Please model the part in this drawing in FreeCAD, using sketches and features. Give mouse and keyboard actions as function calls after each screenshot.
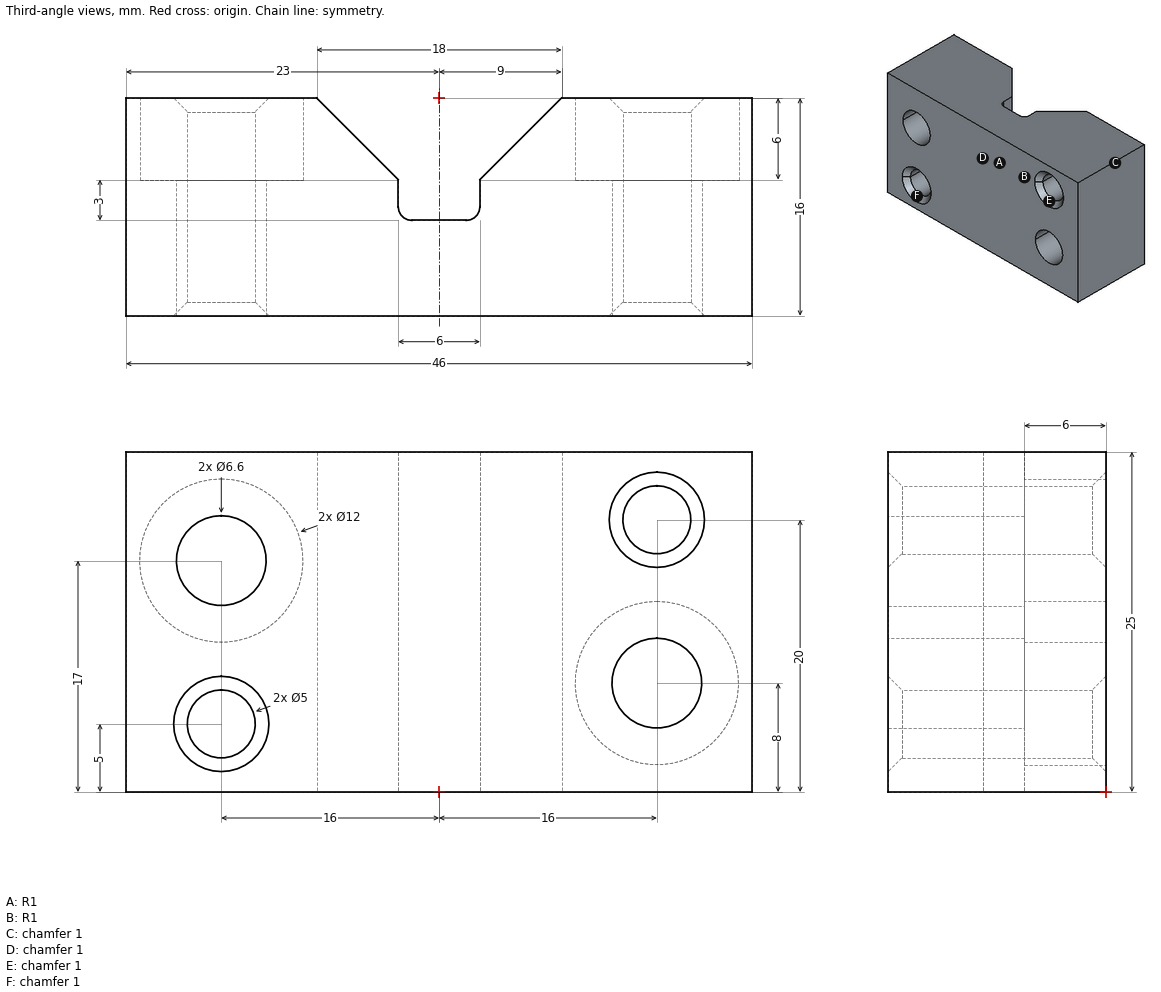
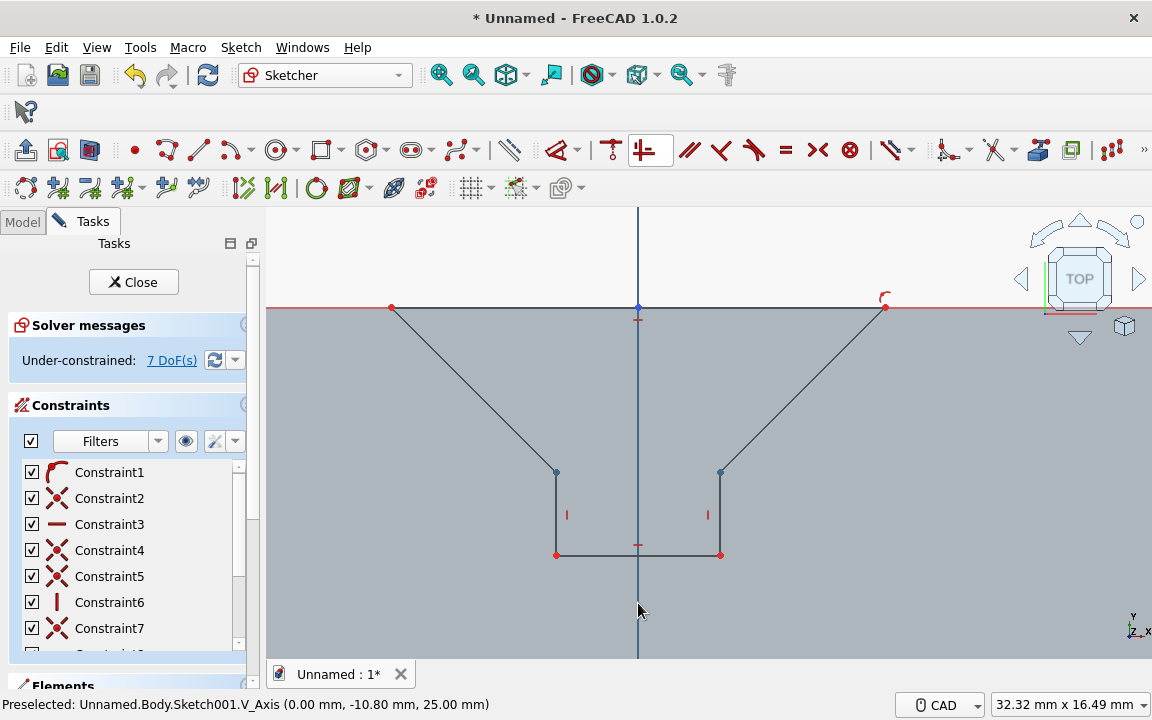
click(818, 150)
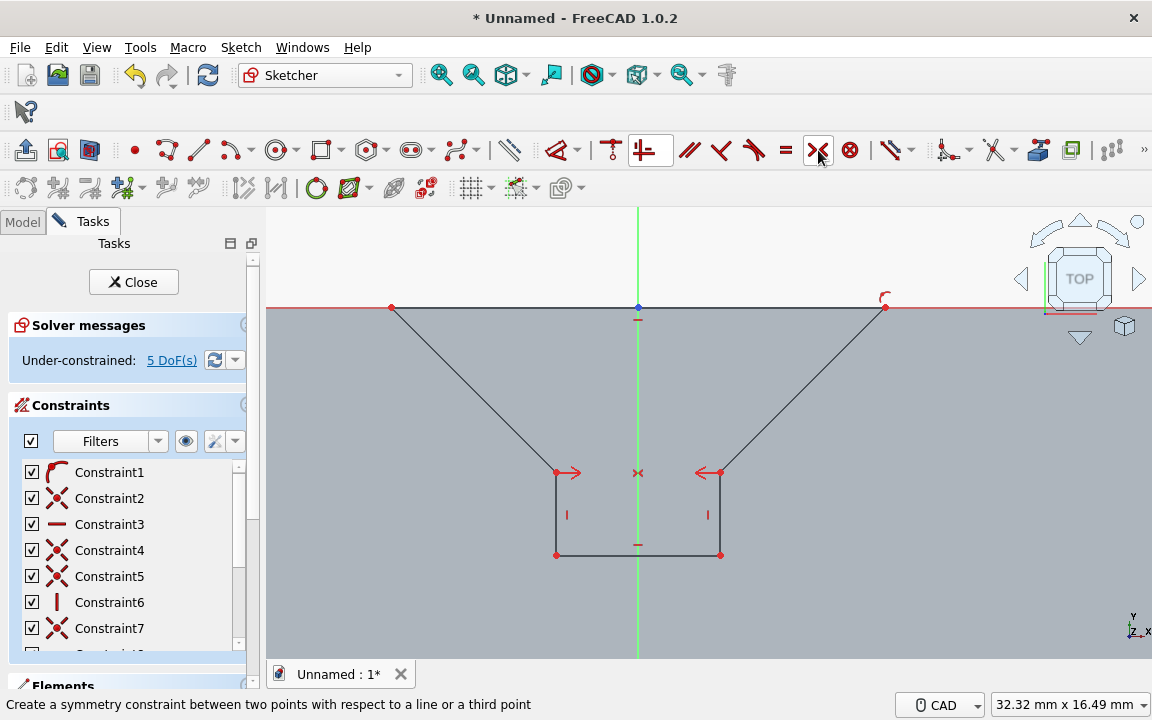
click(556, 498)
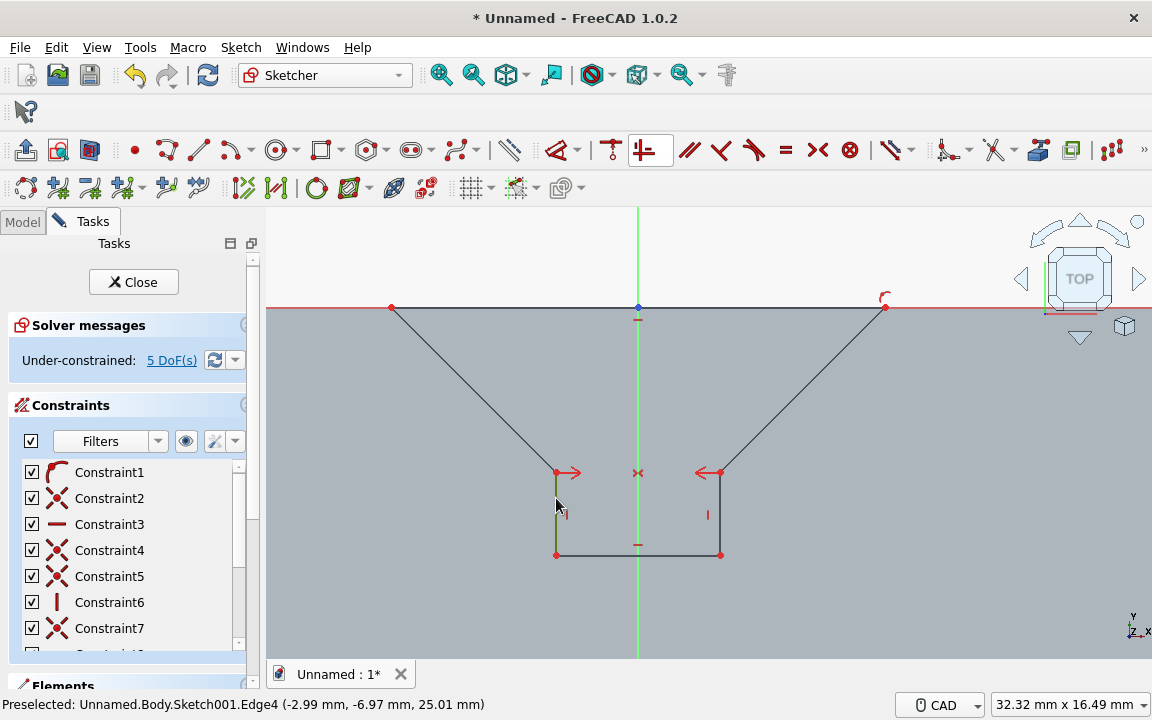
key(i)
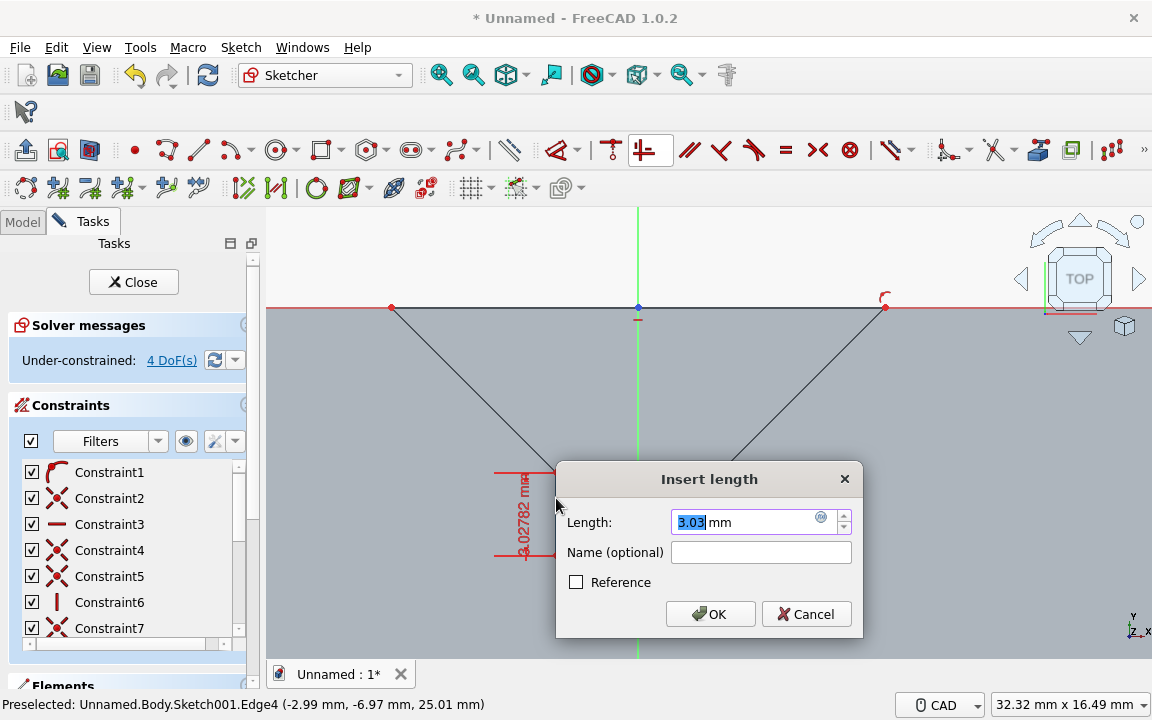
text(3)
key(Return)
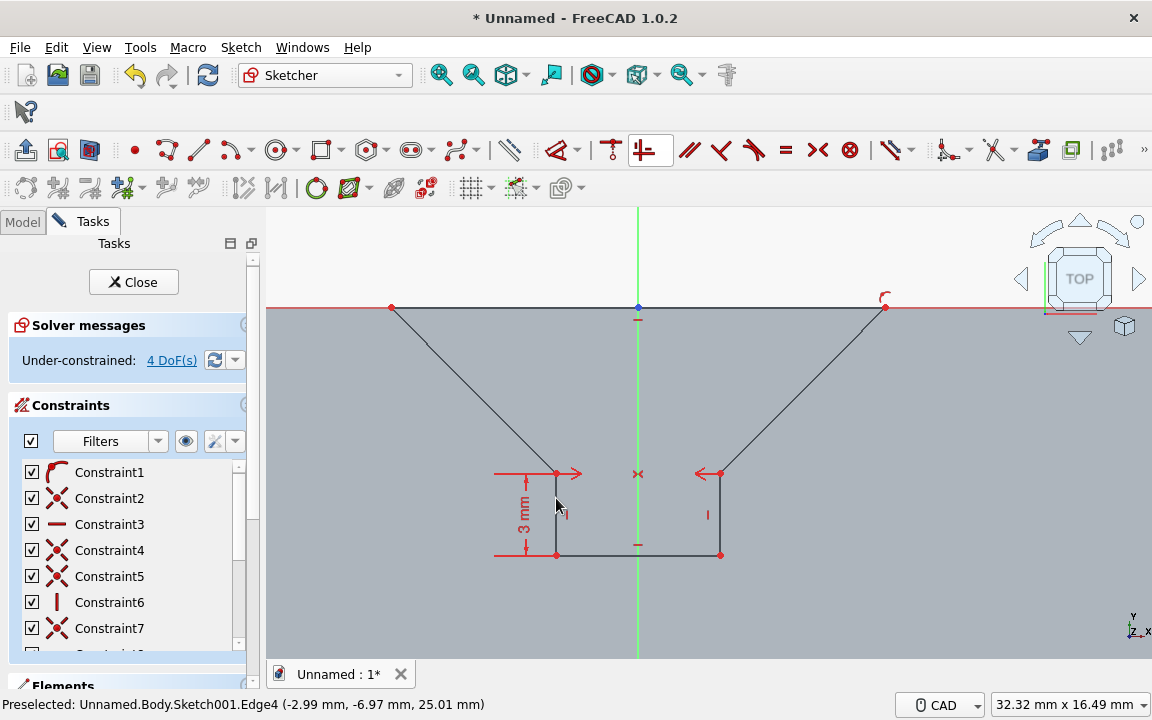
click(605, 556)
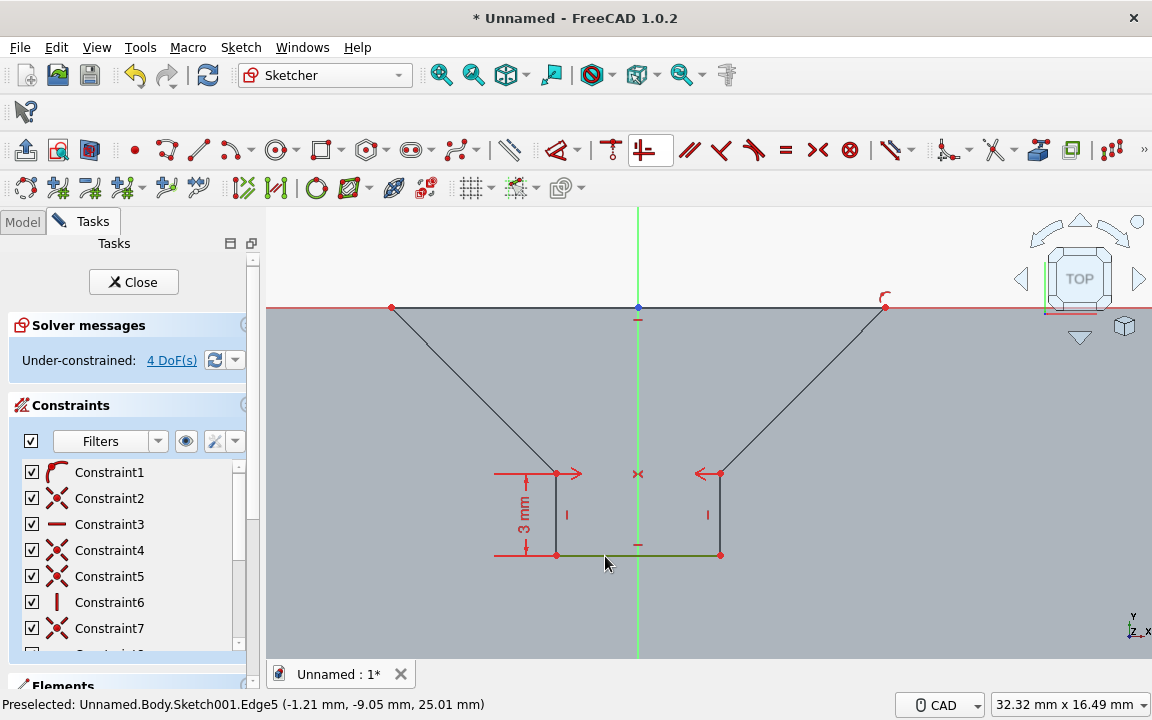
key(l)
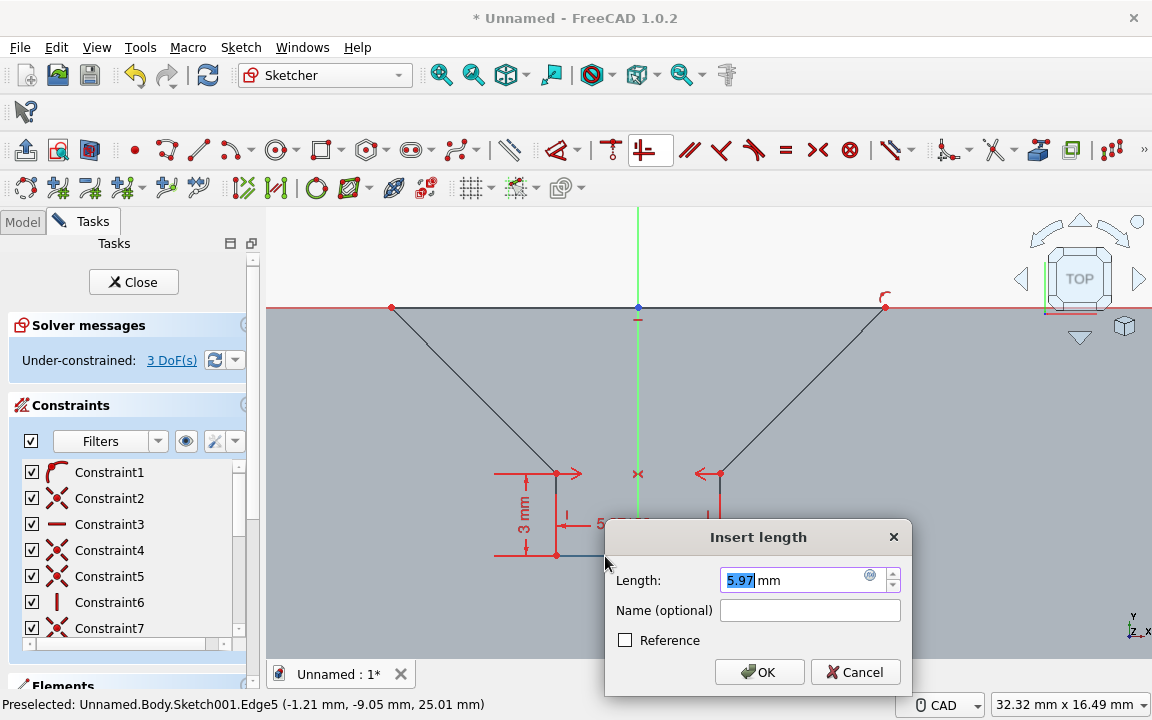
text(6)
key(Return)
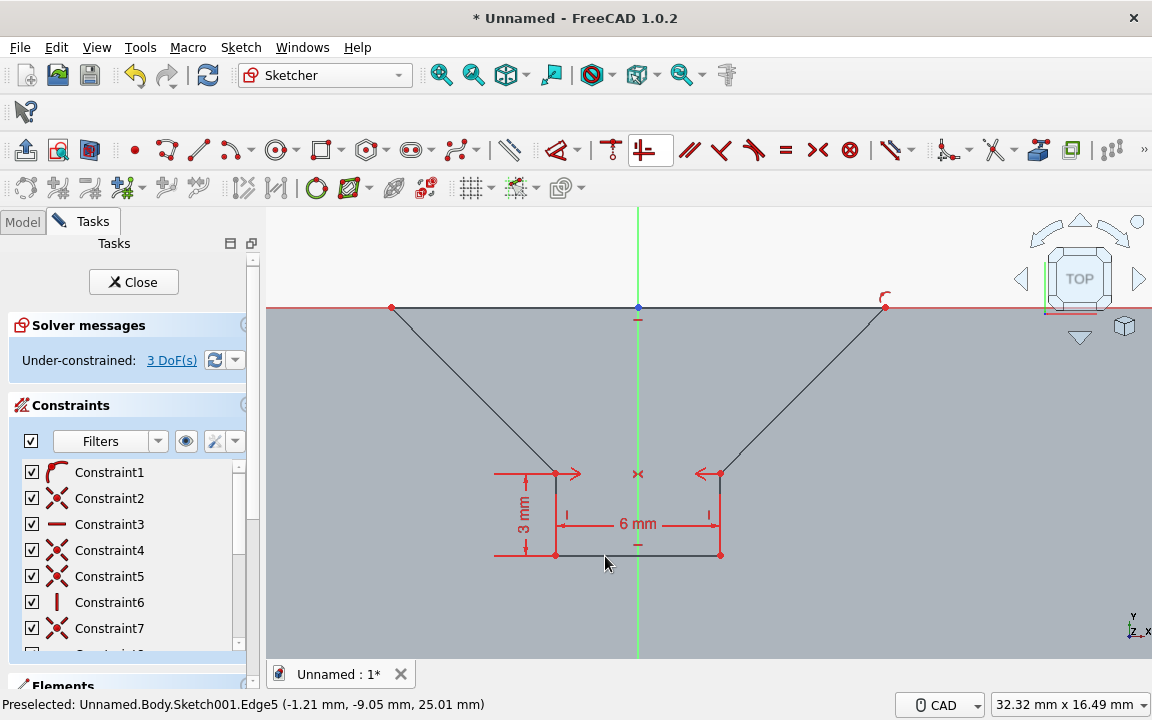
click(737, 308)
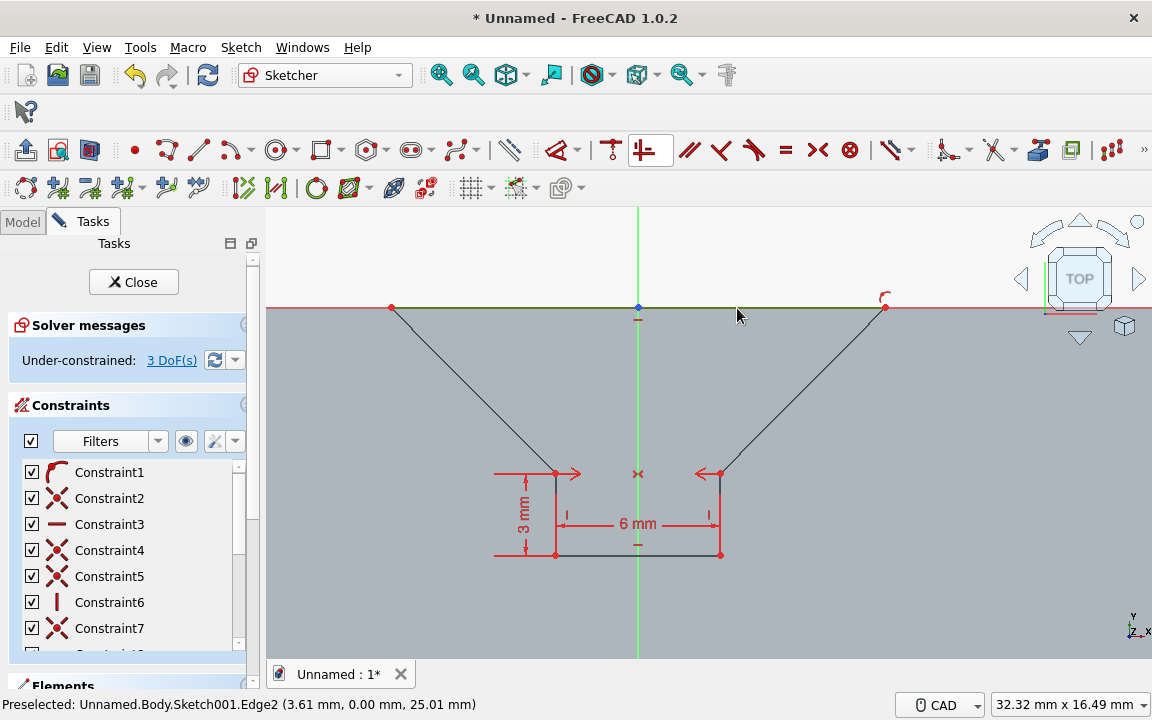
key(l)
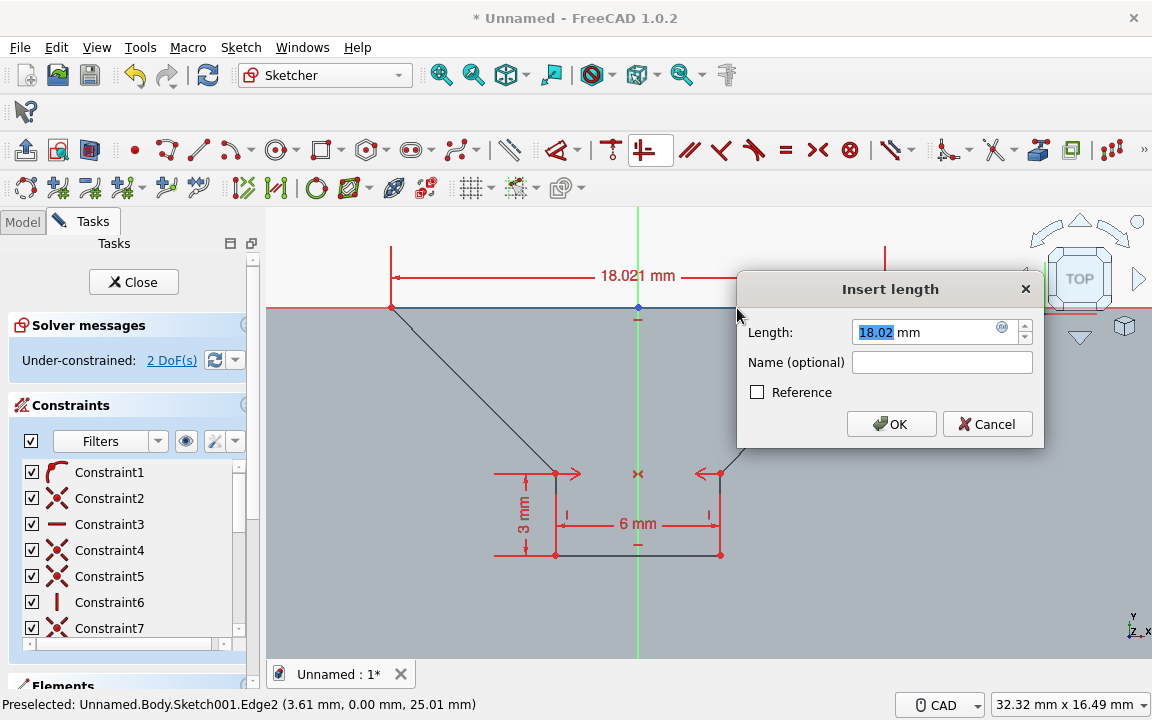
text(18)
key(Return)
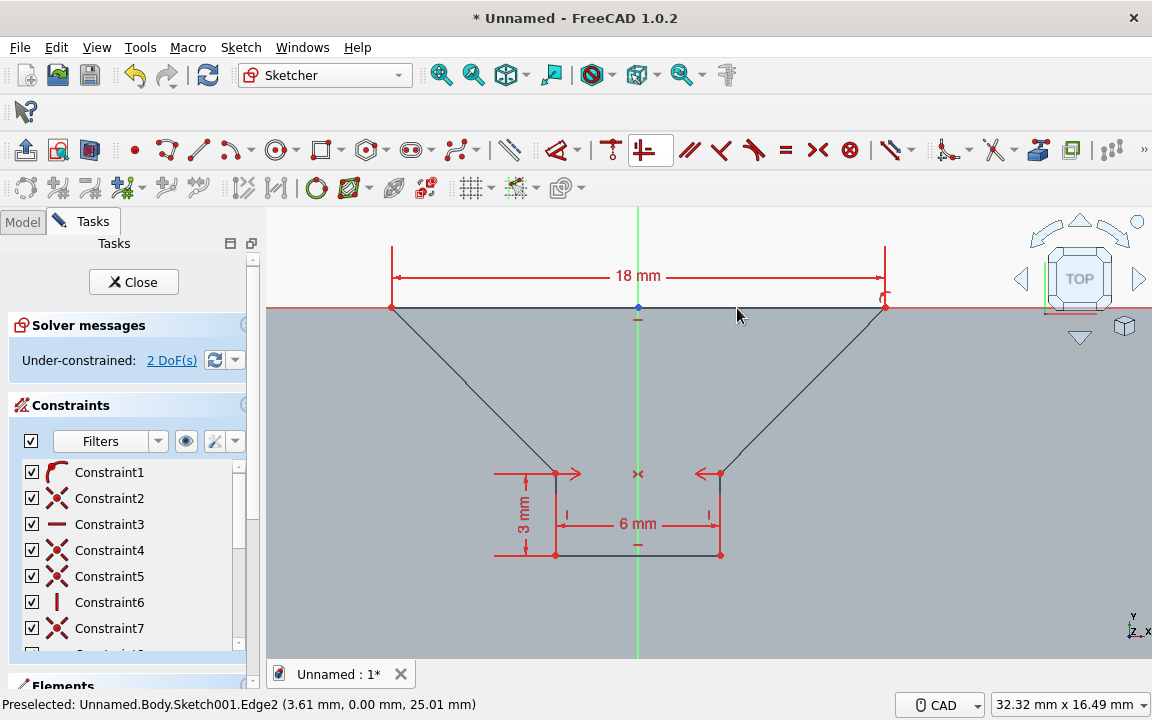
click(720, 474)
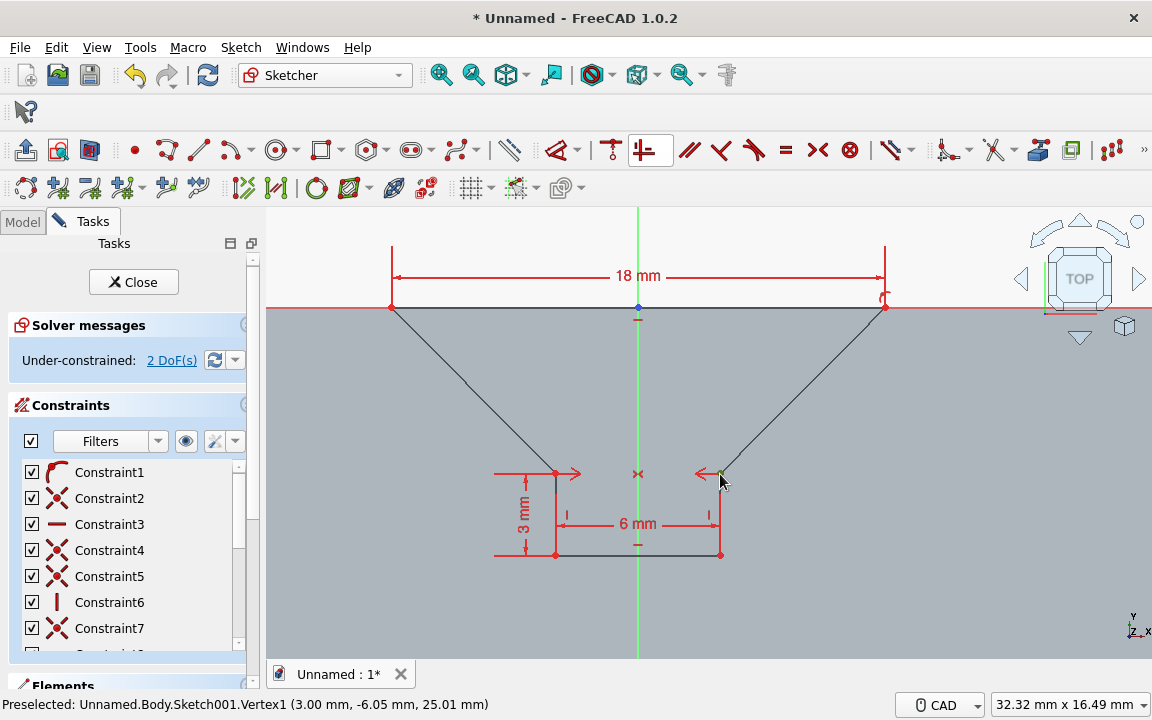
key(i)